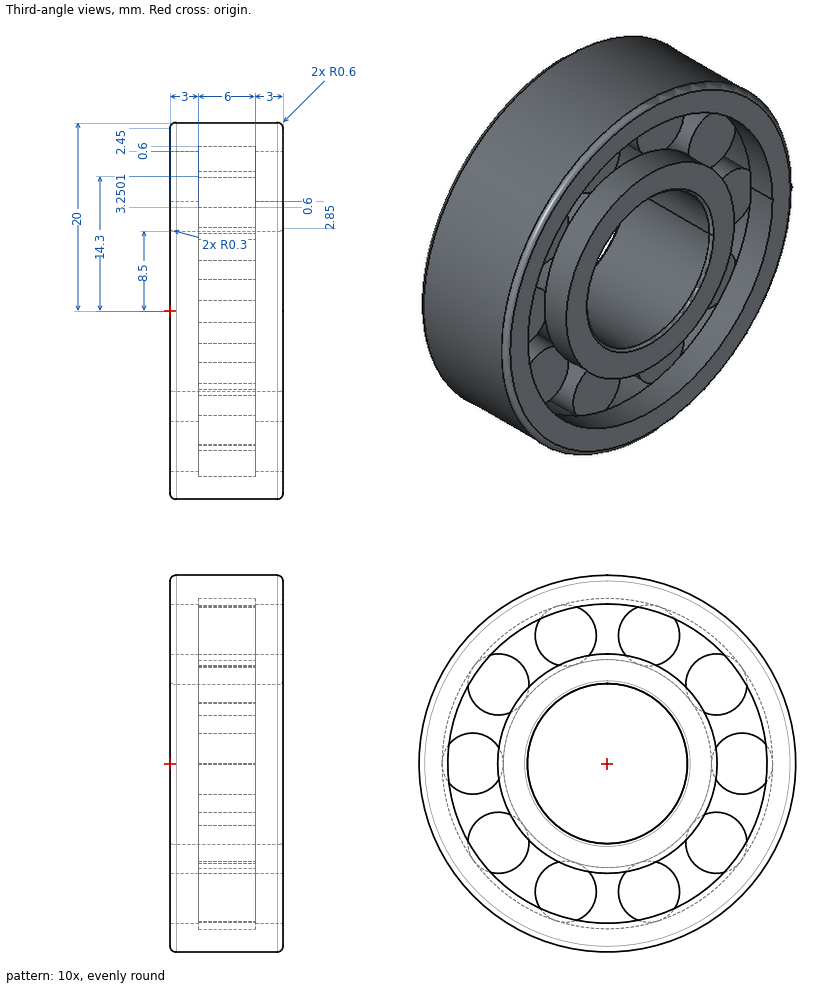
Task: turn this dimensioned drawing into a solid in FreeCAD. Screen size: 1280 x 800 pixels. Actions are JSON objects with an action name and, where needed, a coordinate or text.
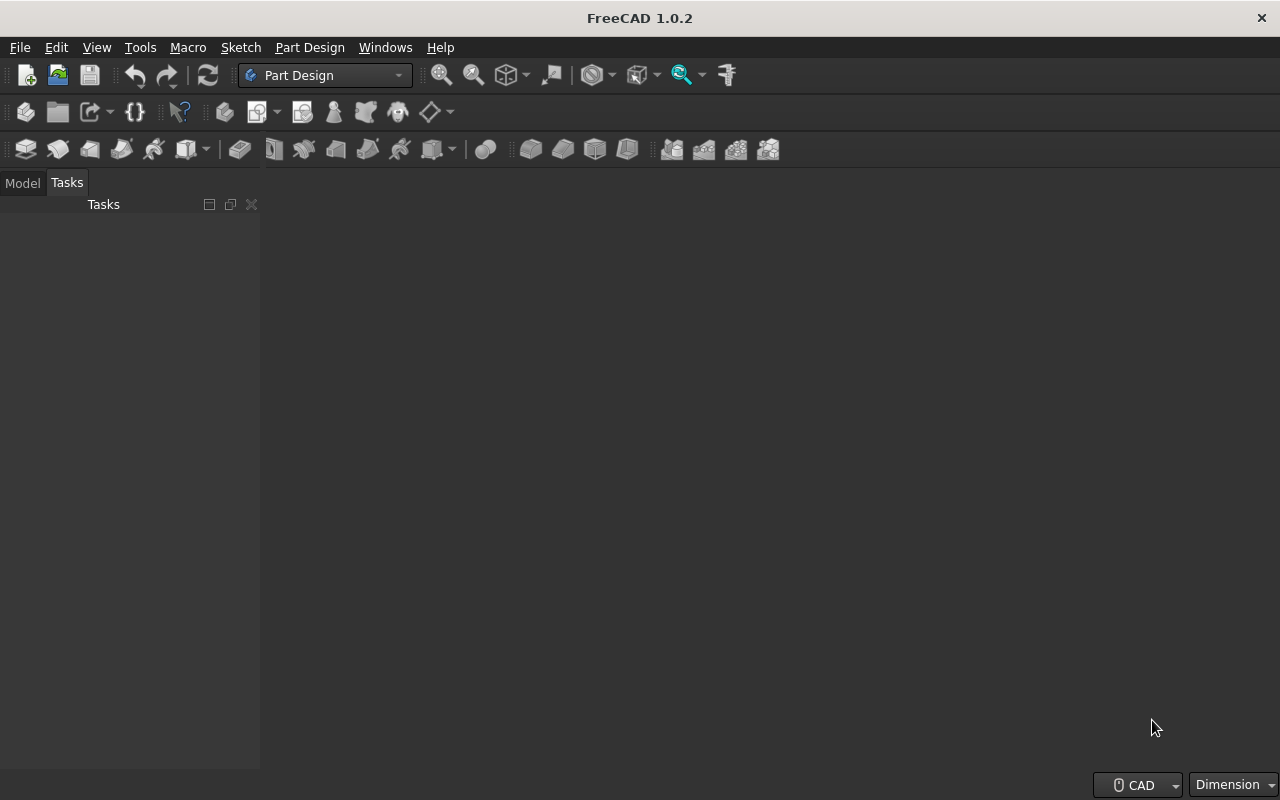
{"action": "left_click", "coordinate": [216, 112]}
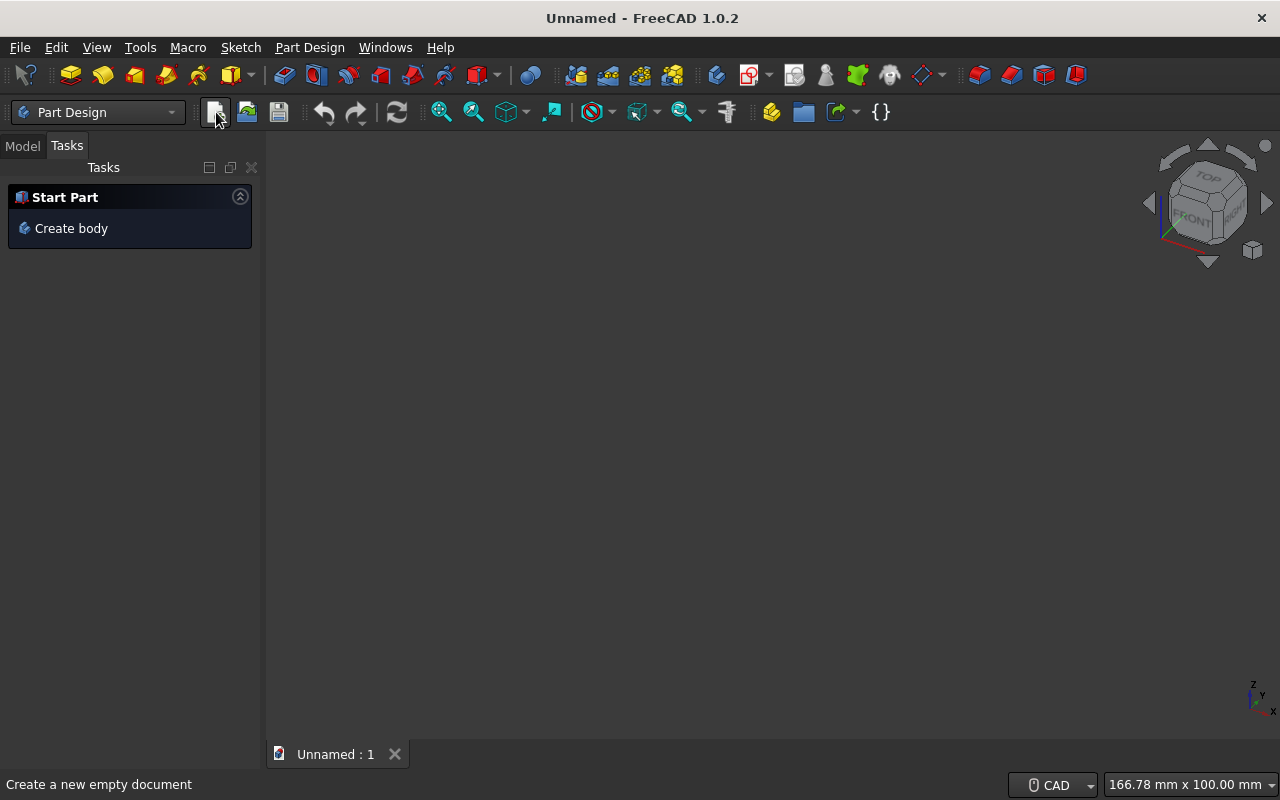
{"action": "left_click", "coordinate": [750, 76]}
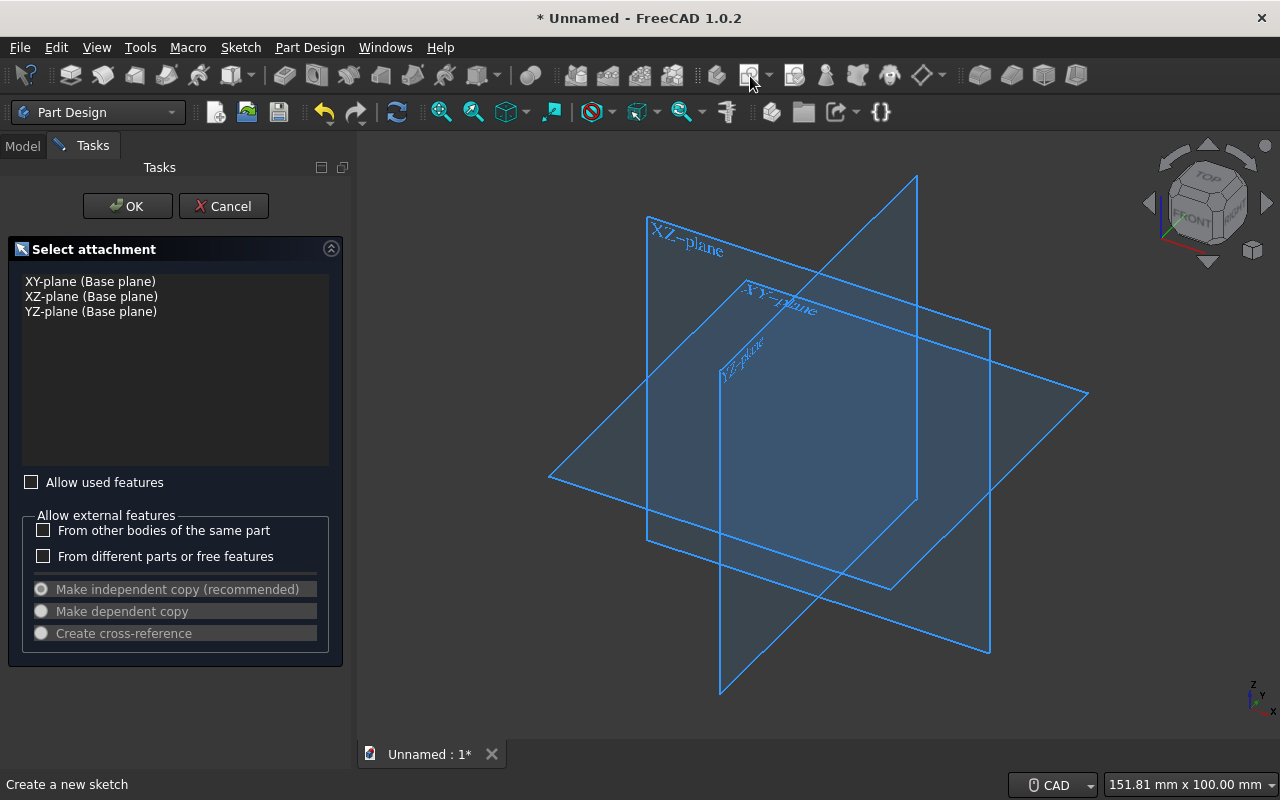
{"action": "left_click", "coordinate": [82, 282]}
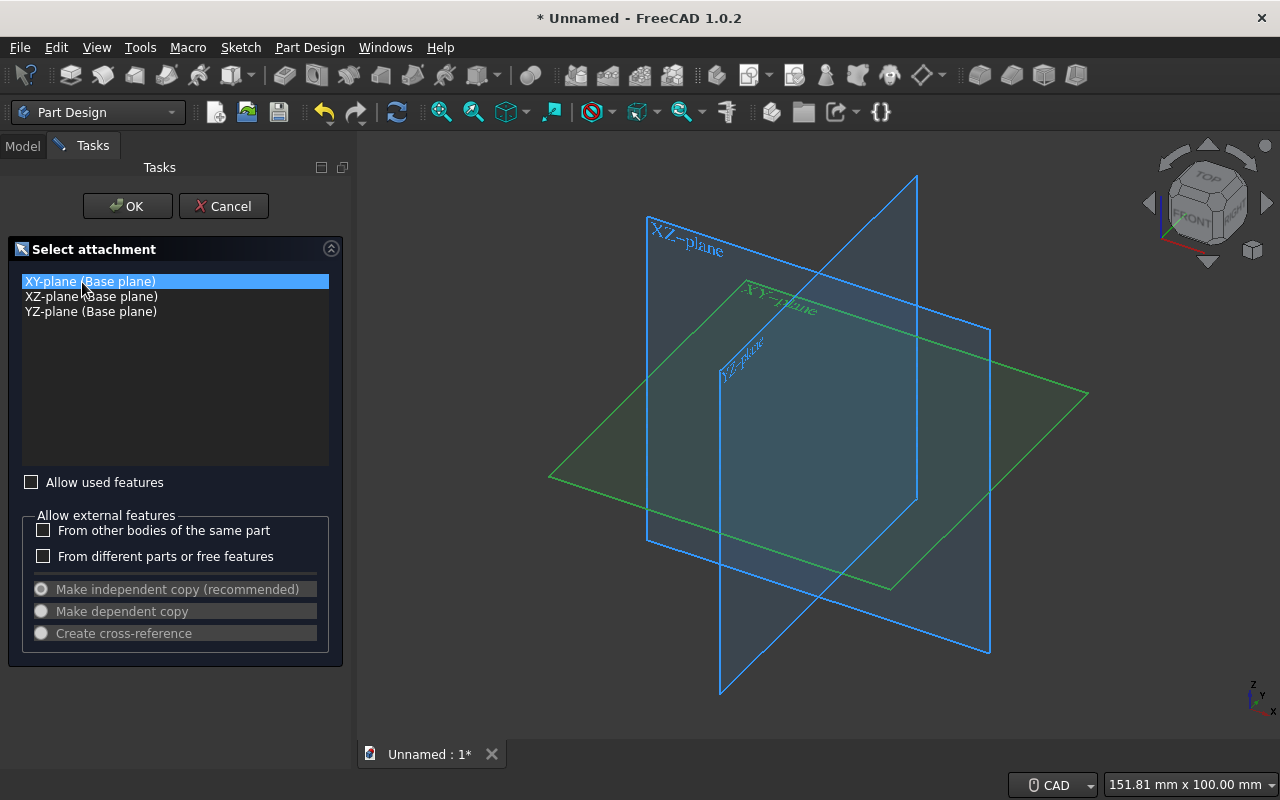
{"action": "left_click", "coordinate": [128, 206]}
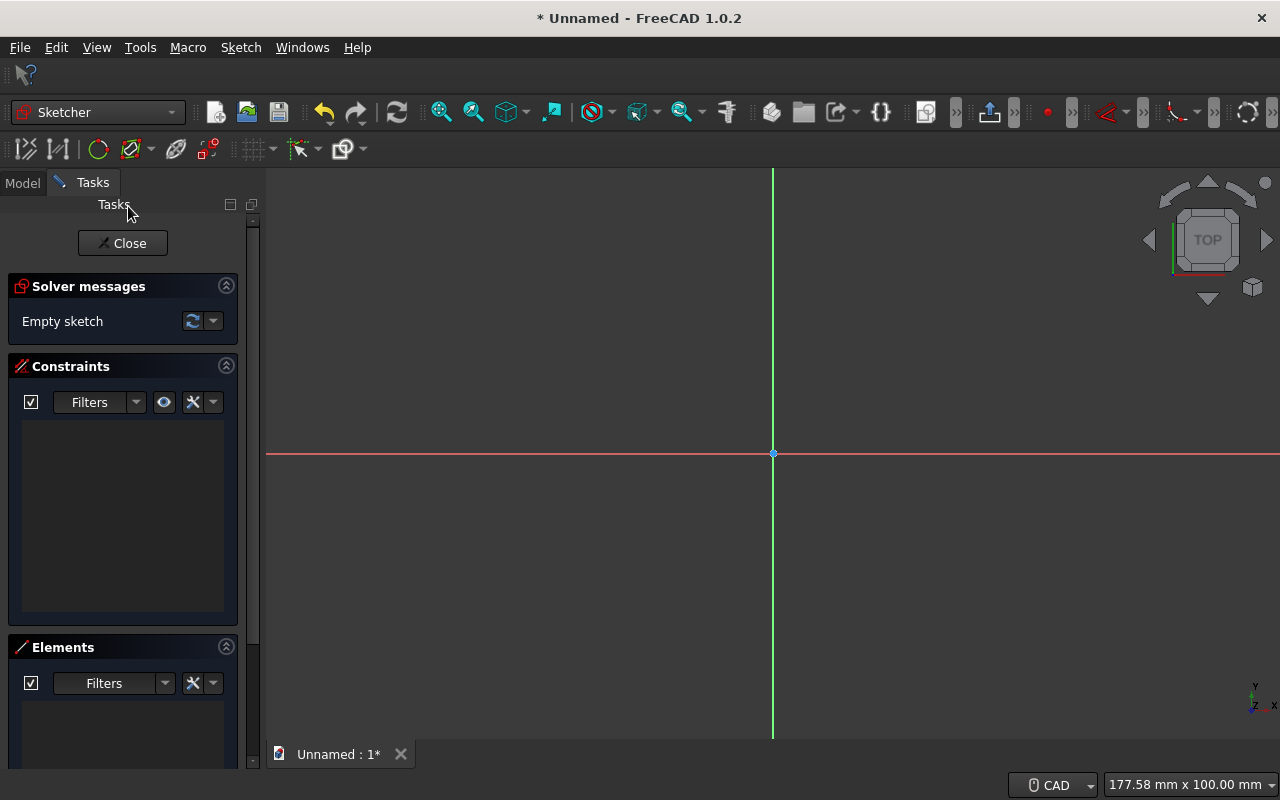
{"action": "scroll", "coordinate": [833, 412], "scroll_direction": "up", "scroll_amount": 8}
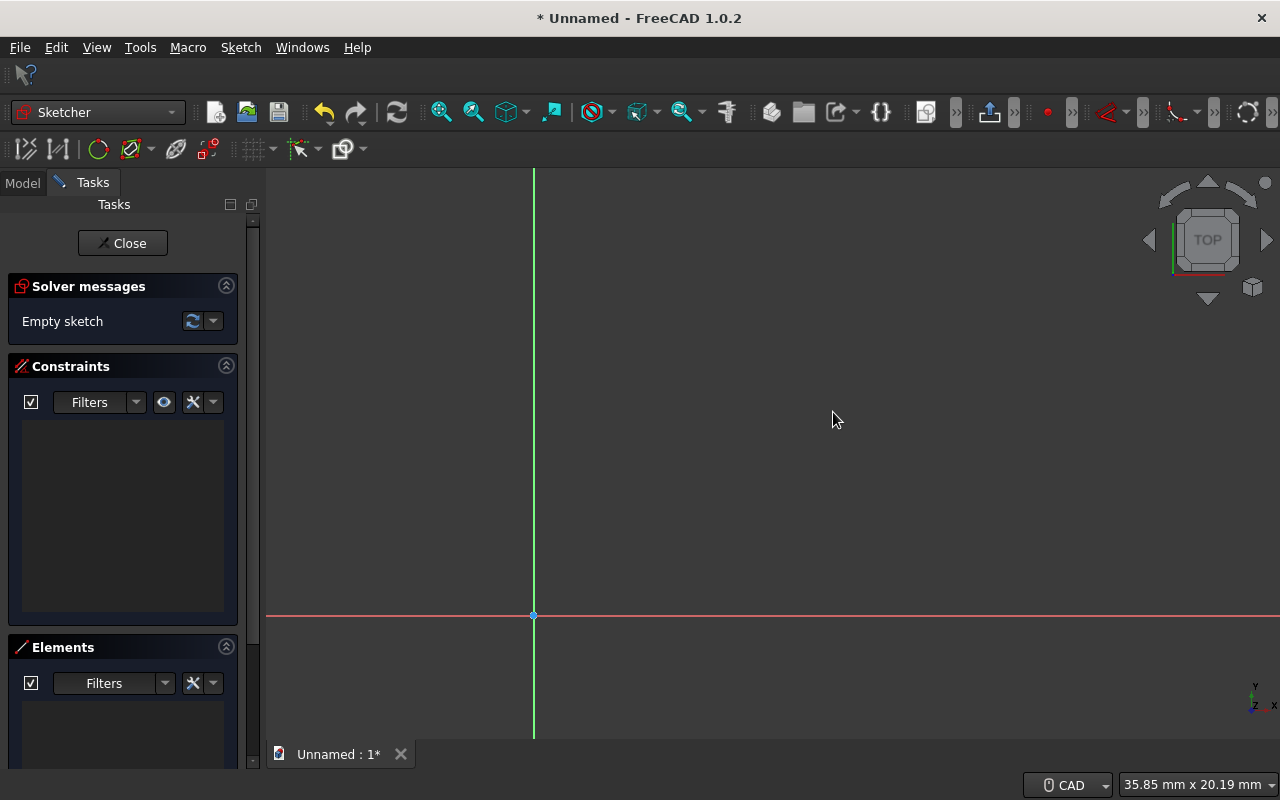
{"action": "key", "text": "g l"}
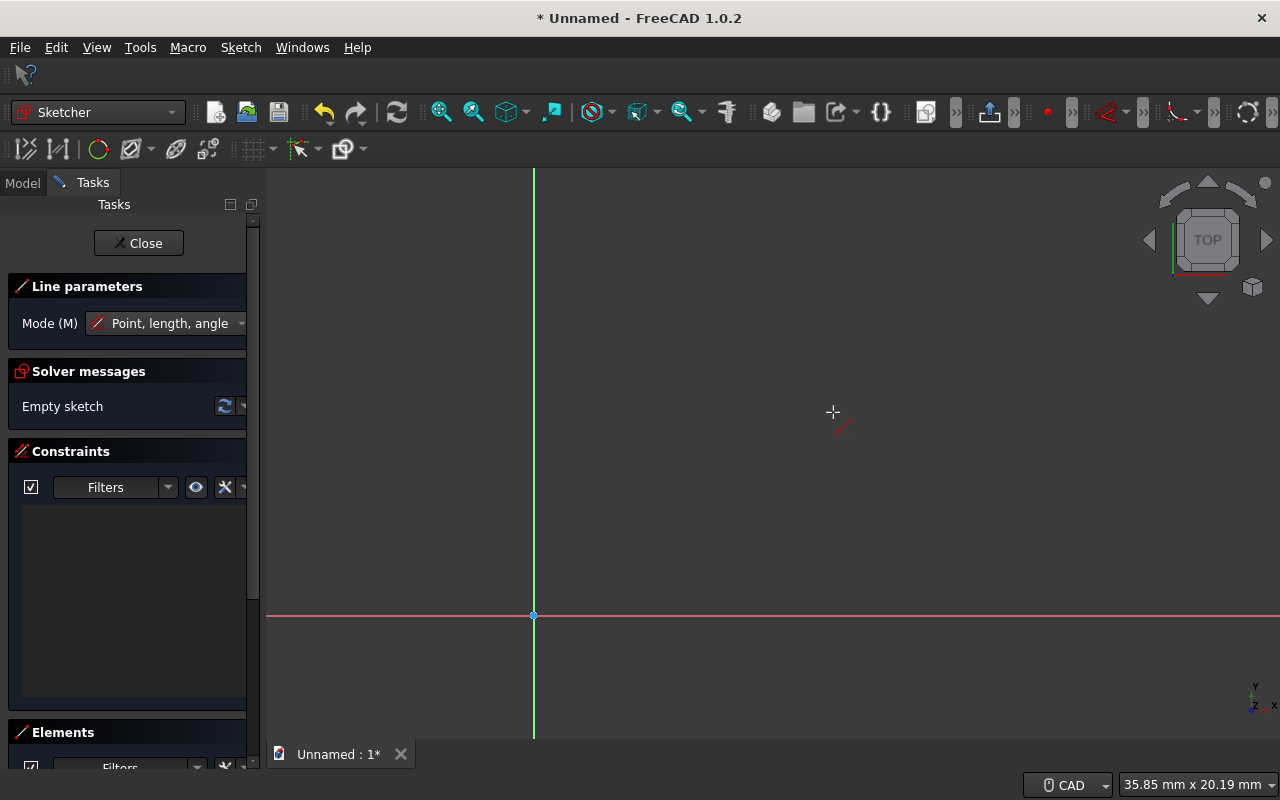
{"action": "scroll", "coordinate": [542, 375], "scroll_direction": "up", "scroll_amount": 4}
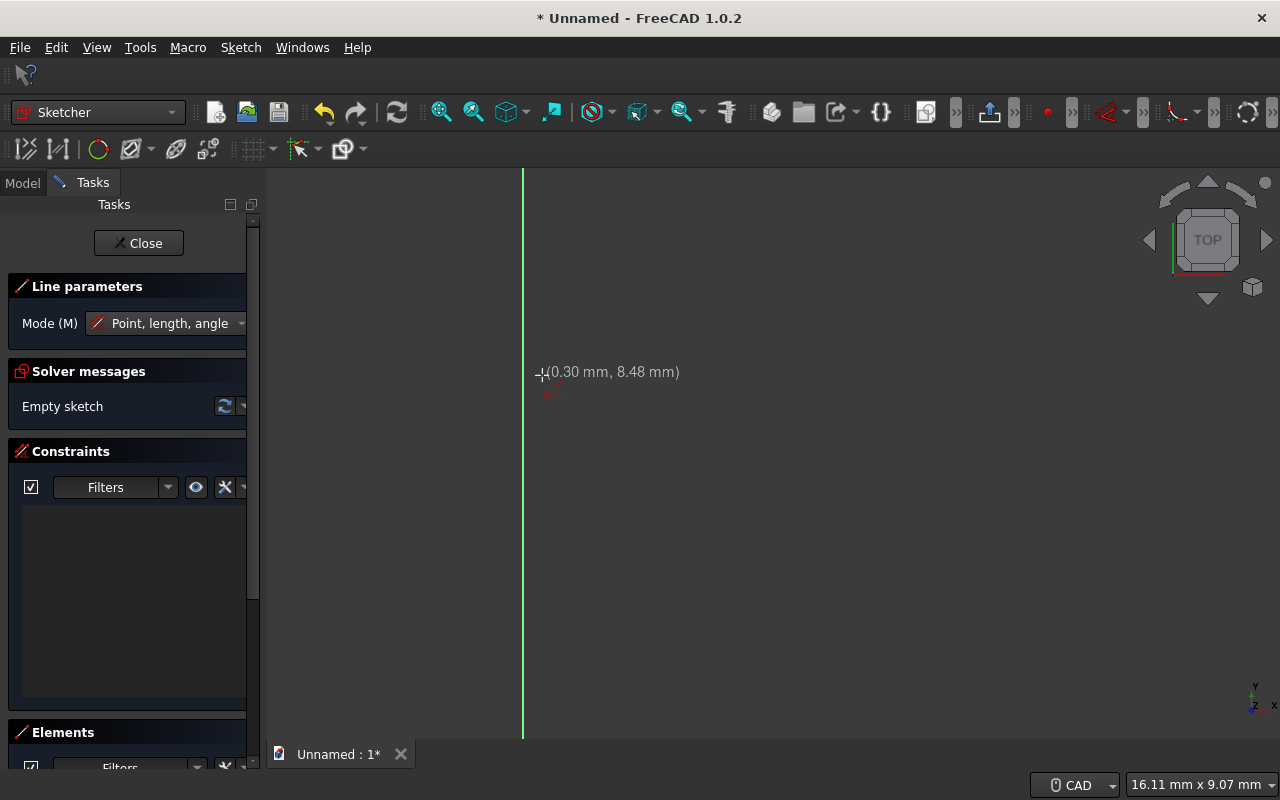
{"action": "left_click", "coordinate": [542, 376]}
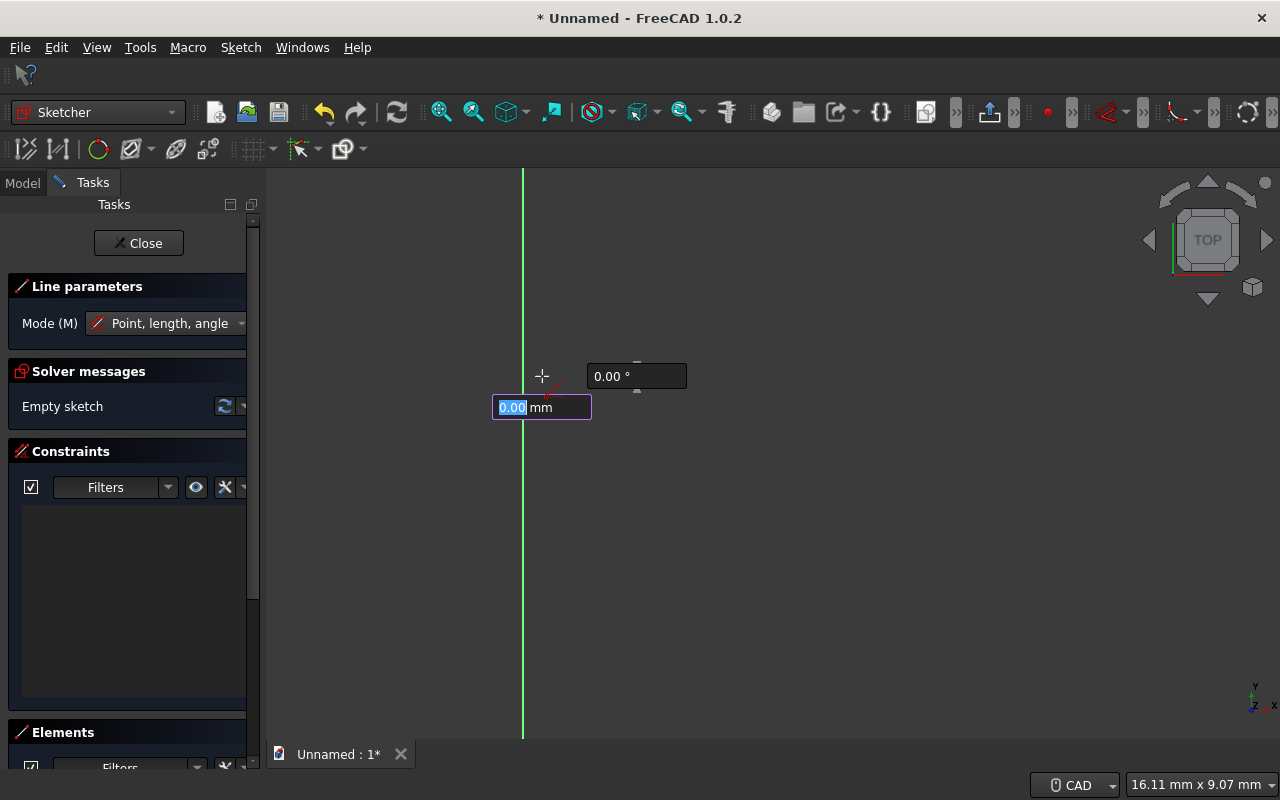
{"action": "scroll", "coordinate": [544, 380], "scroll_direction": "down", "scroll_amount": 4}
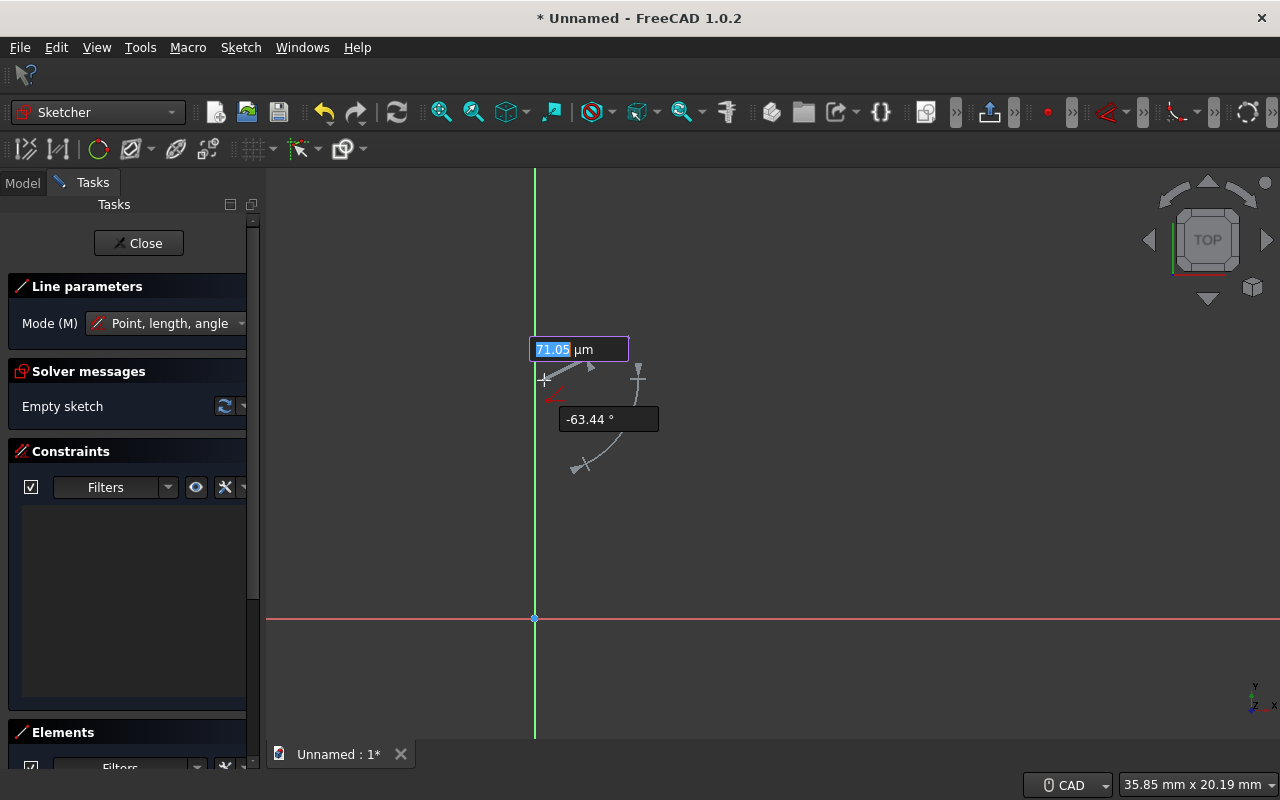
{"action": "left_click", "coordinate": [866, 378]}